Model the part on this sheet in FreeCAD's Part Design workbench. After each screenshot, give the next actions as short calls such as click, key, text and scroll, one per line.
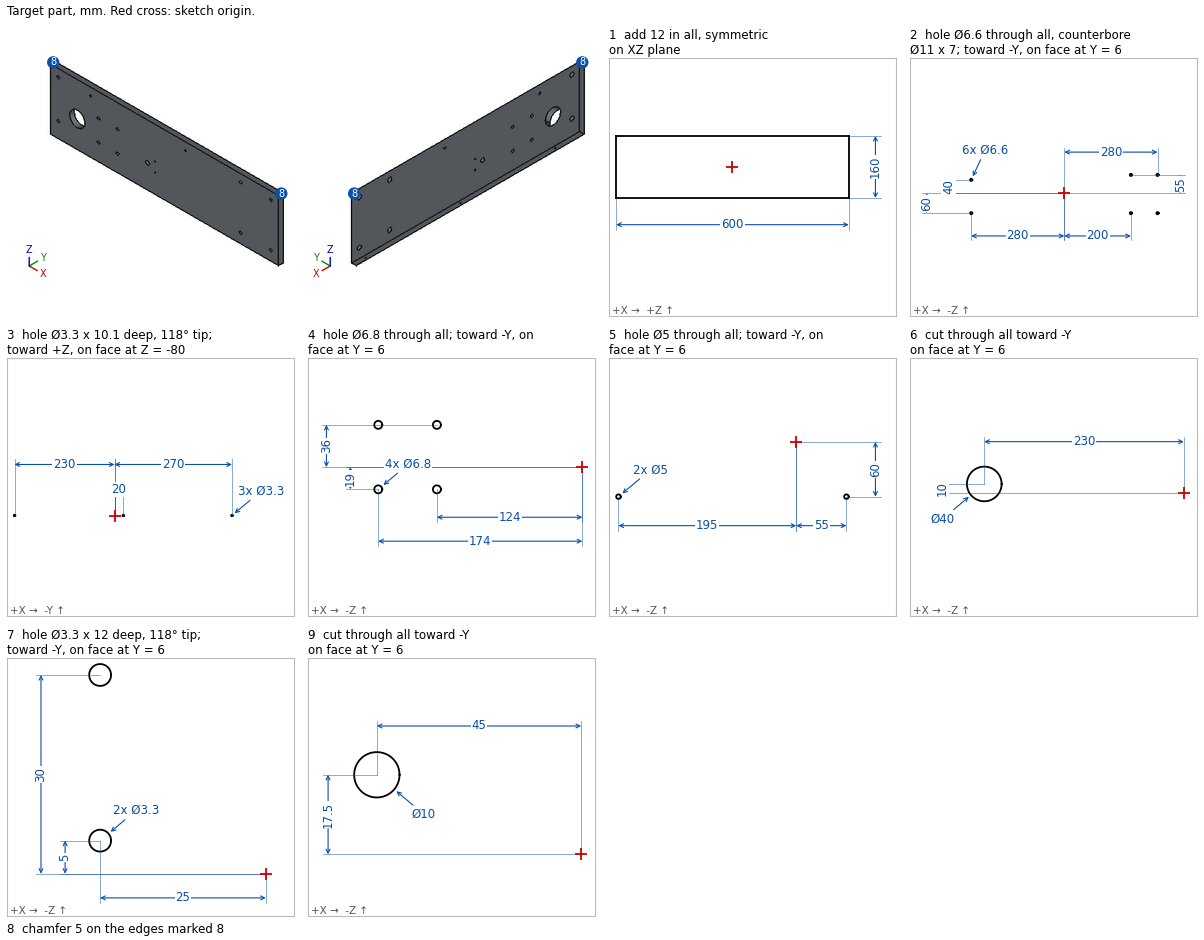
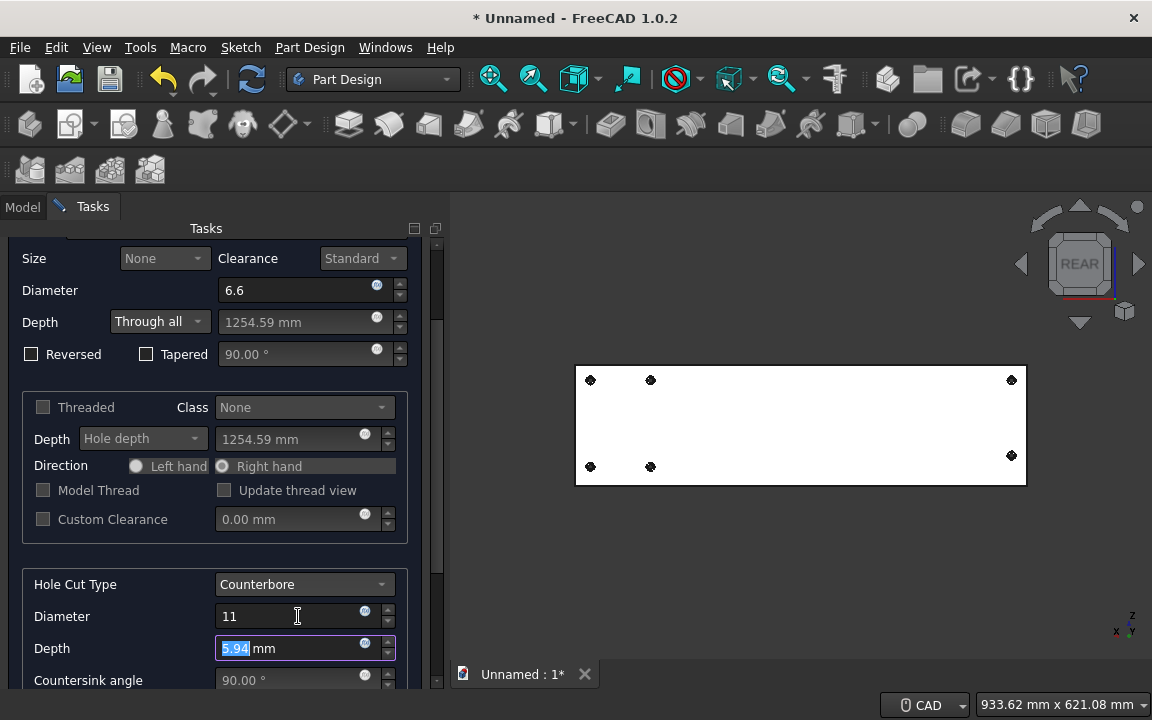
text(7)
key(Tab)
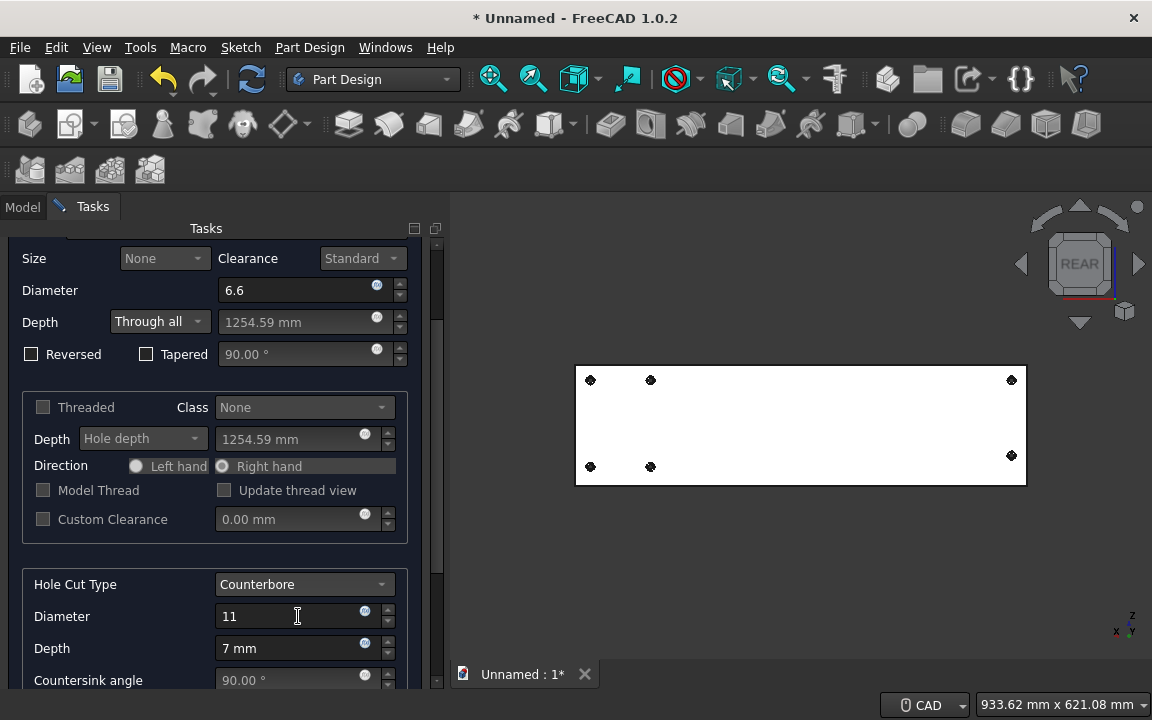
scroll(437, 463, up, 3)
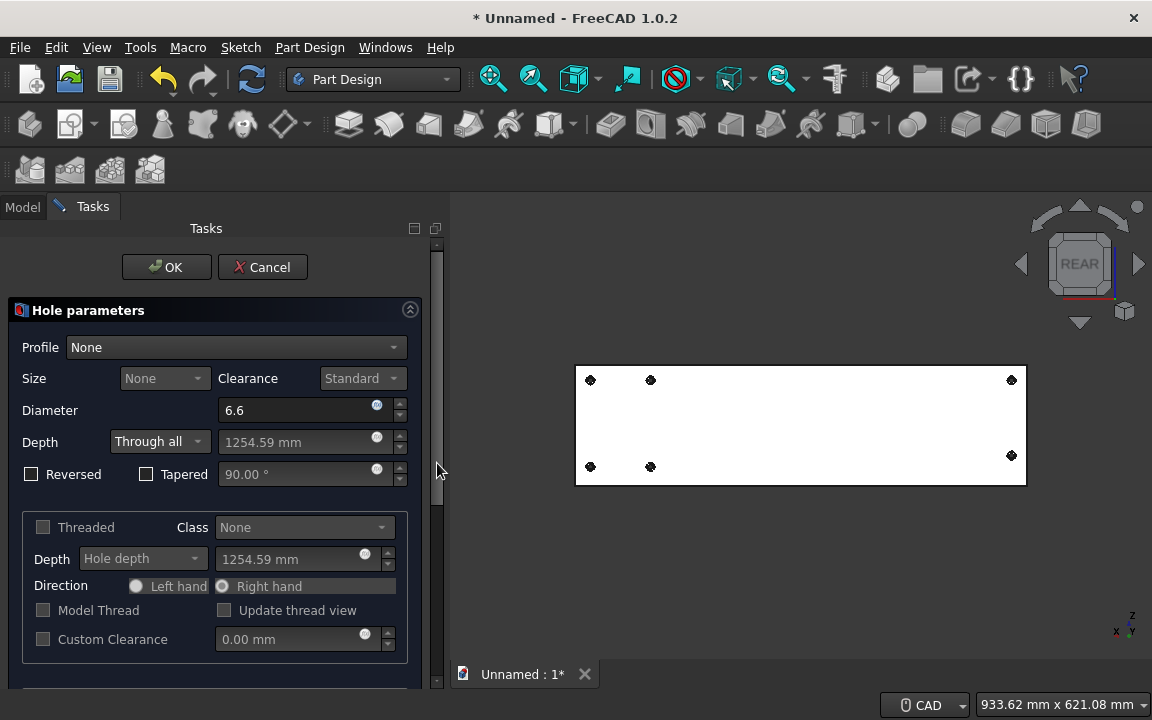
click(167, 267)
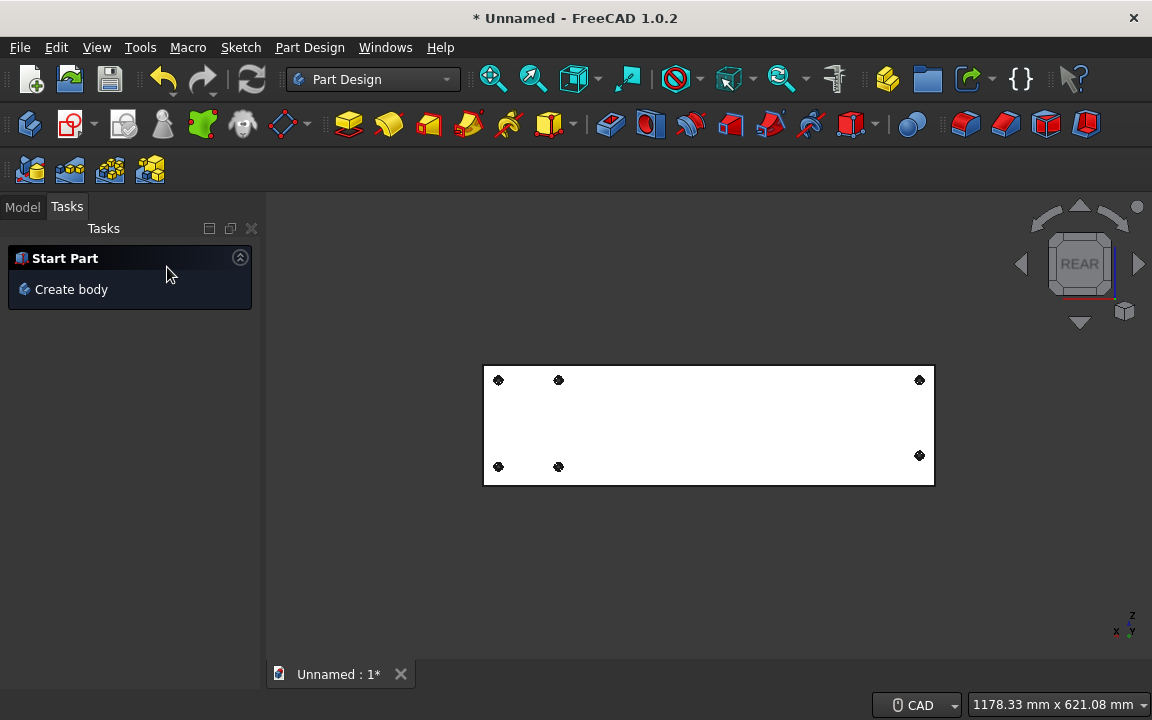
key(5)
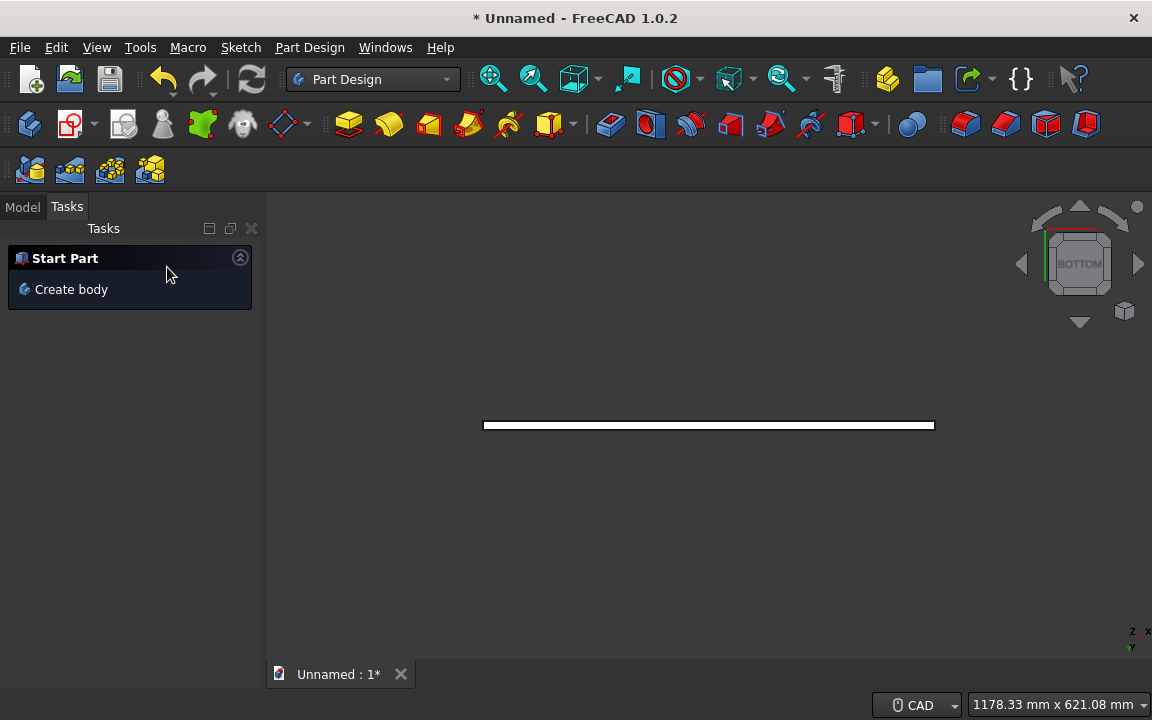
scroll(902, 425, up, 5)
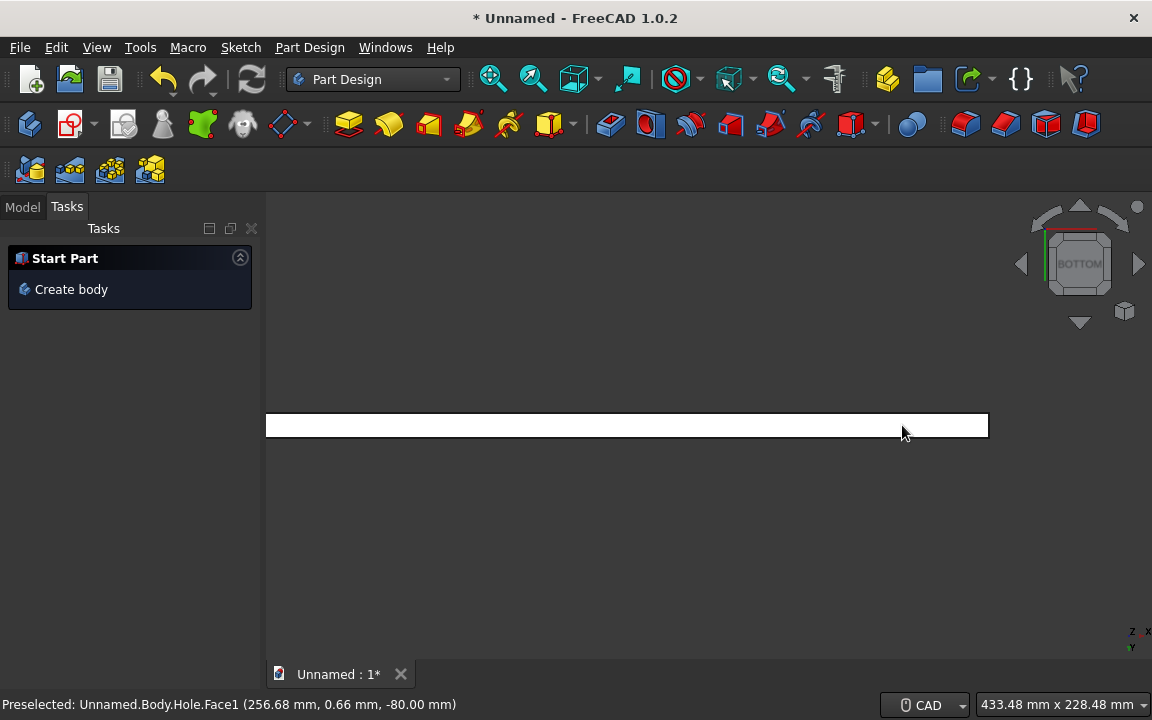
click(902, 425)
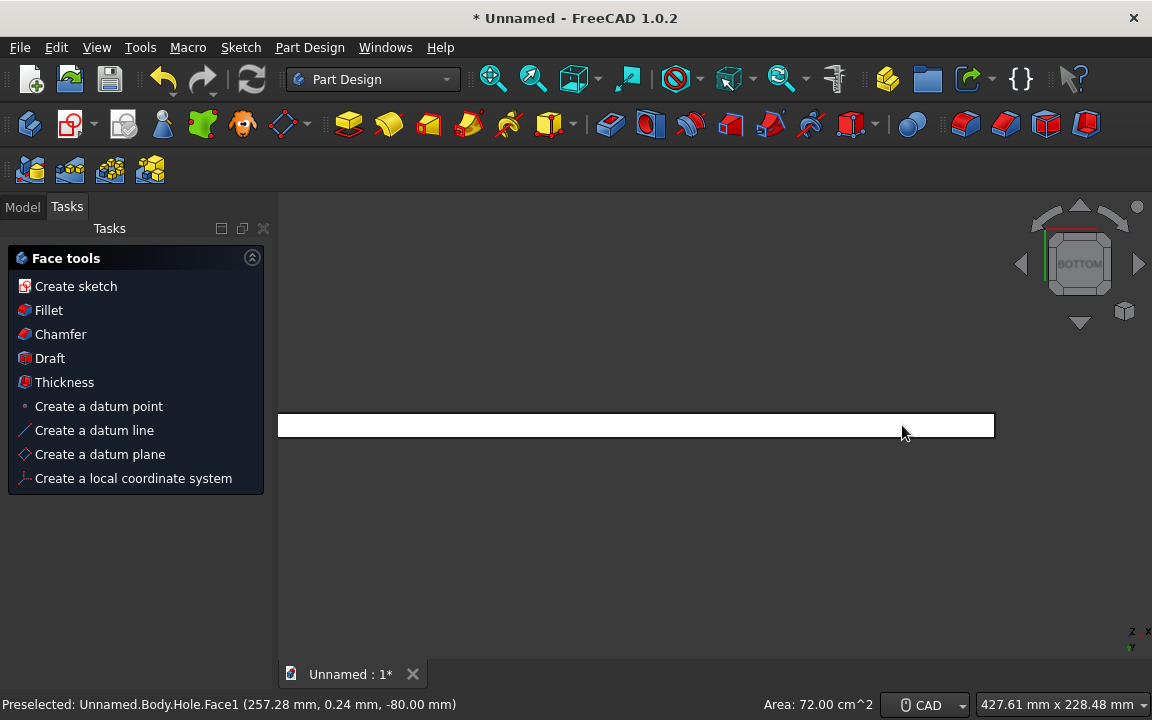
click(70, 124)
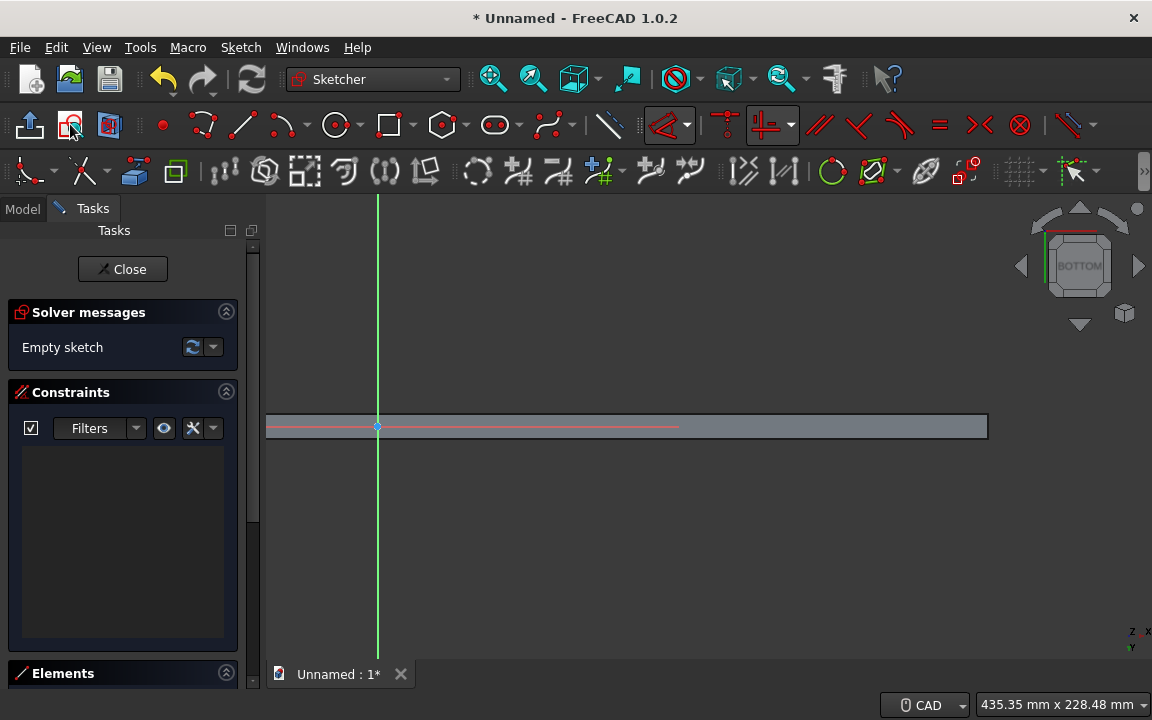
scroll(822, 426, down, 4)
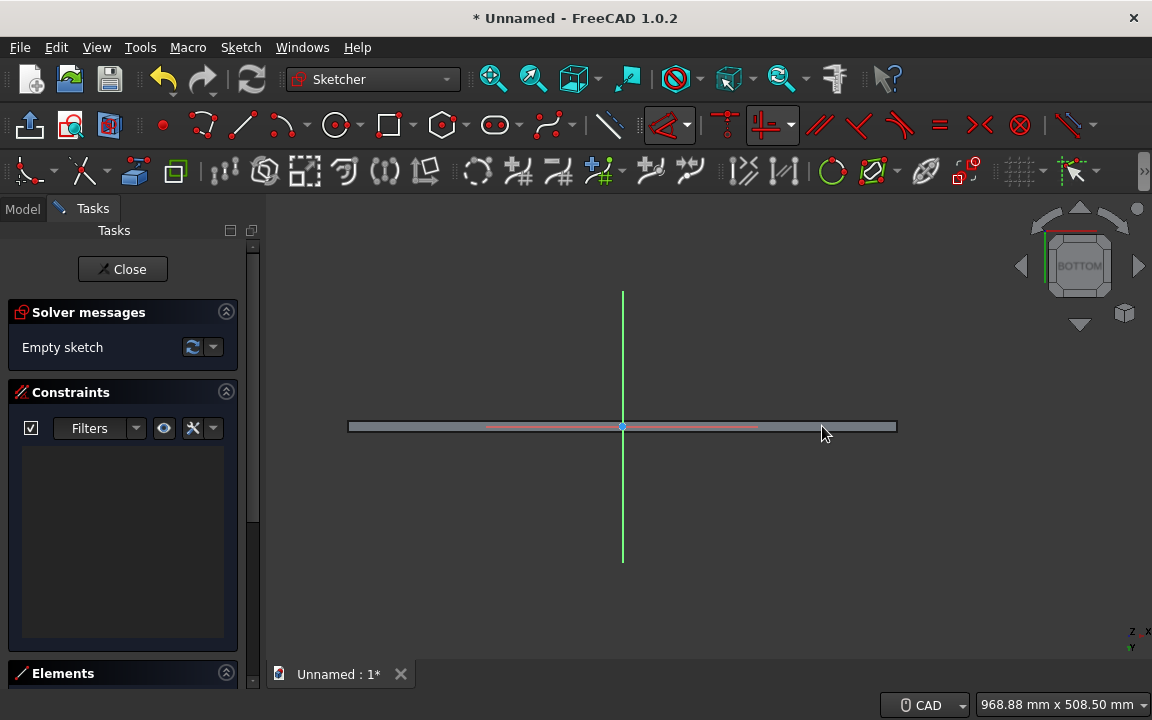
key(g)
key(c)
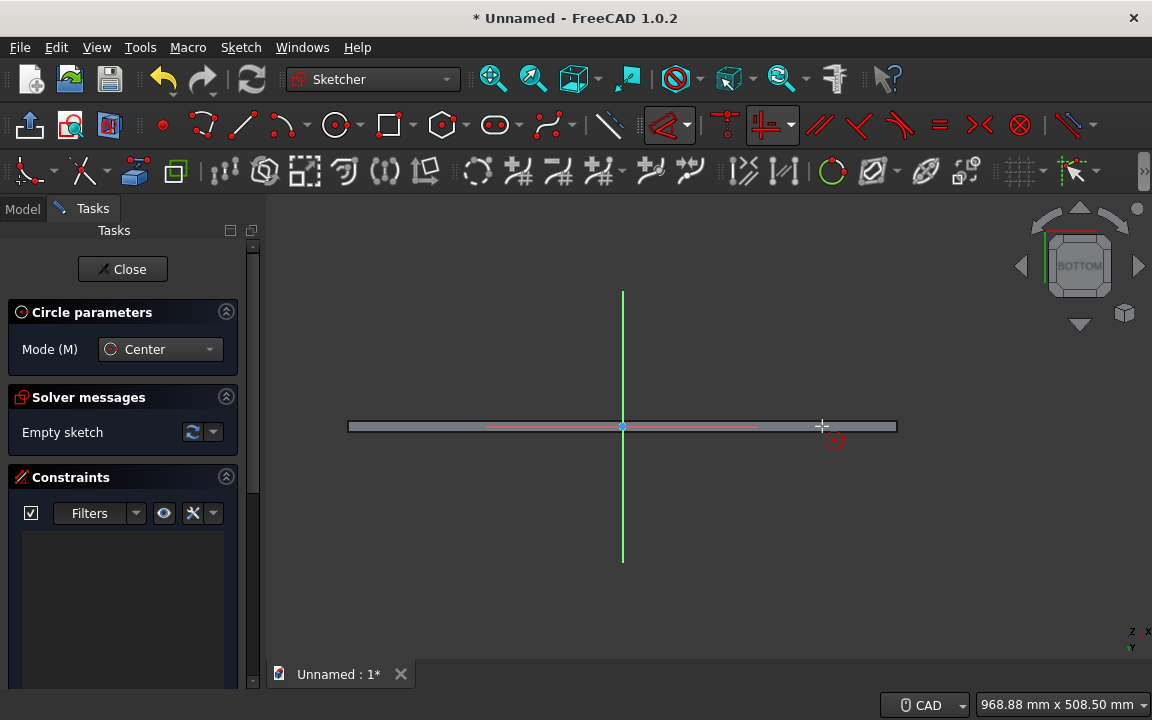
scroll(870, 427, up, 14)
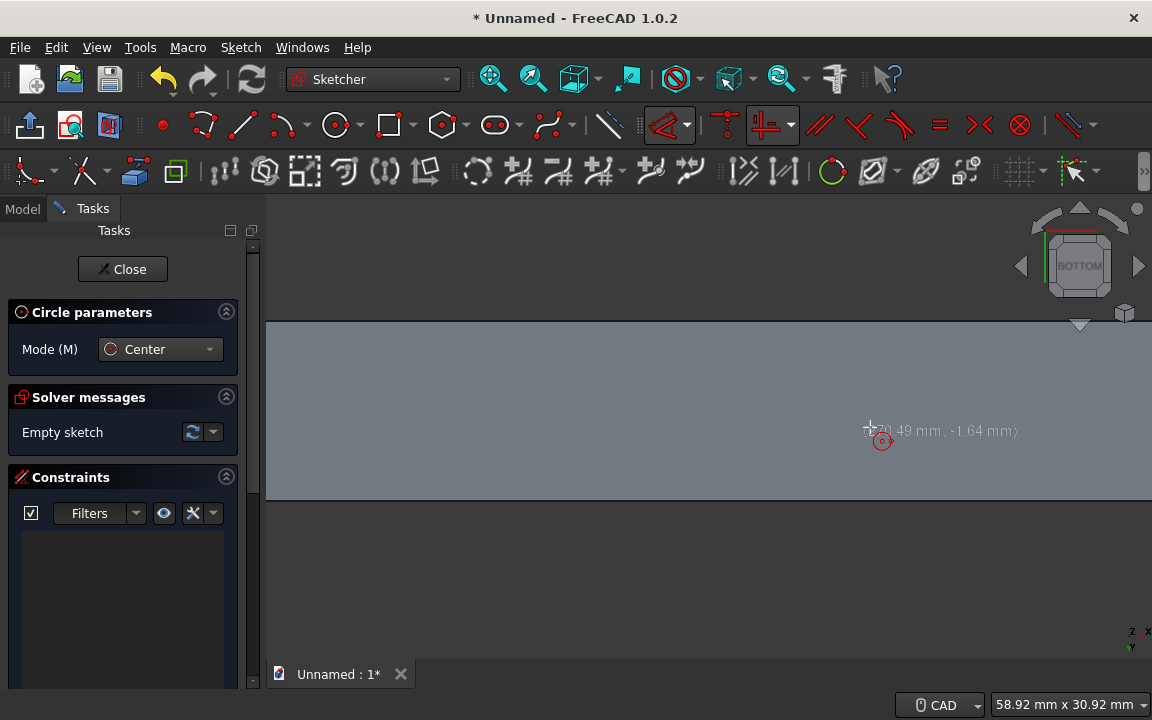
scroll(870, 428, down, 14)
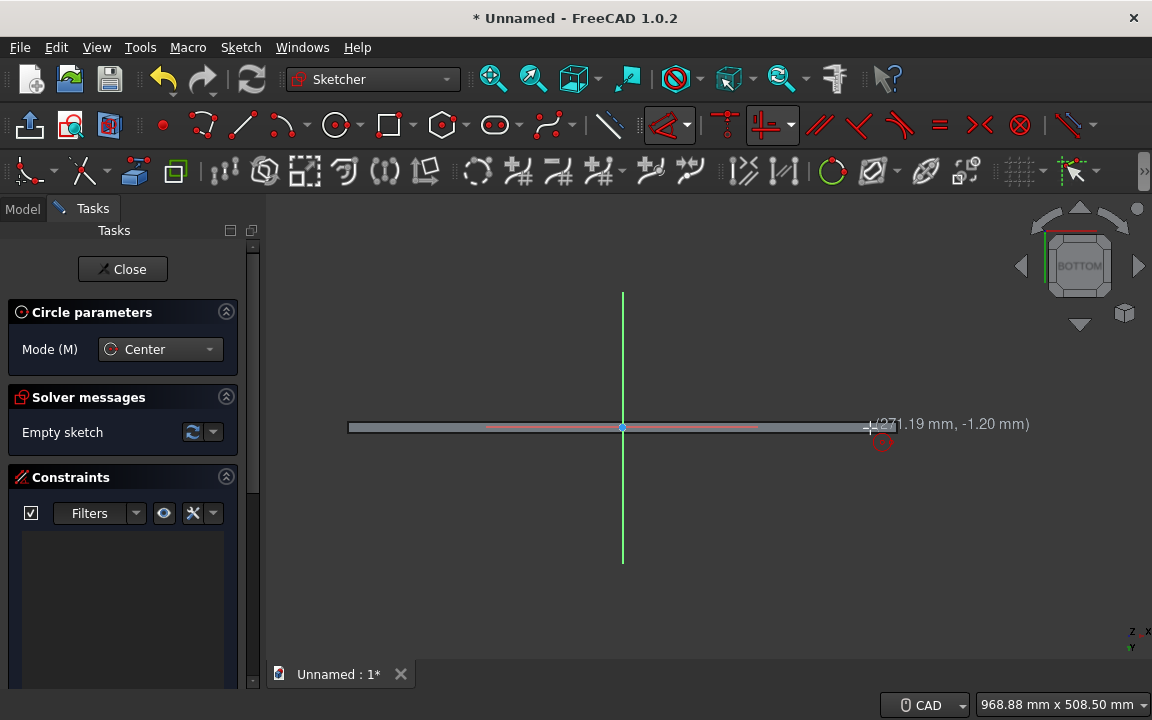
click(870, 427)